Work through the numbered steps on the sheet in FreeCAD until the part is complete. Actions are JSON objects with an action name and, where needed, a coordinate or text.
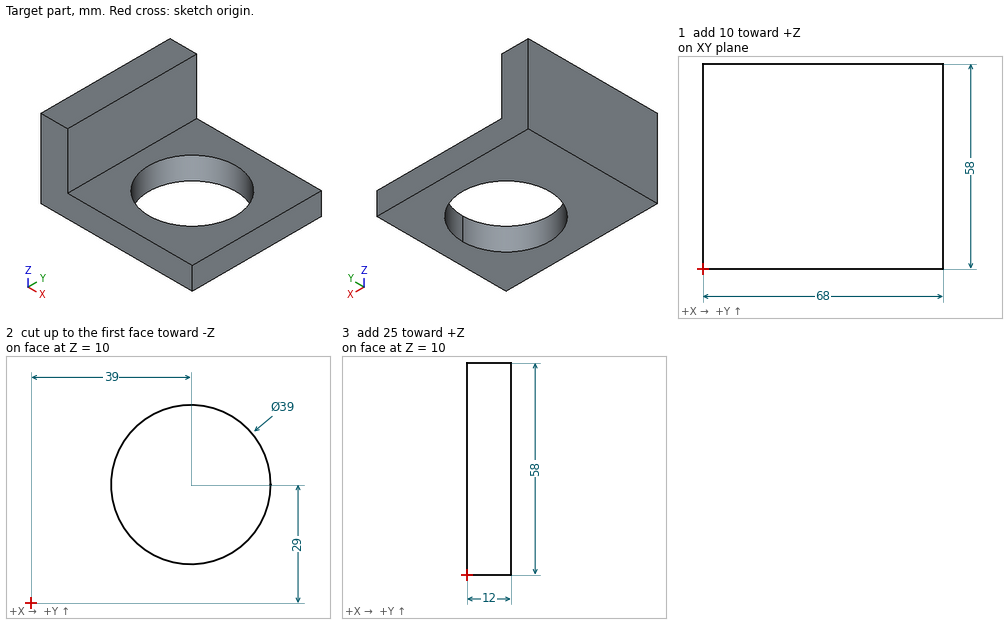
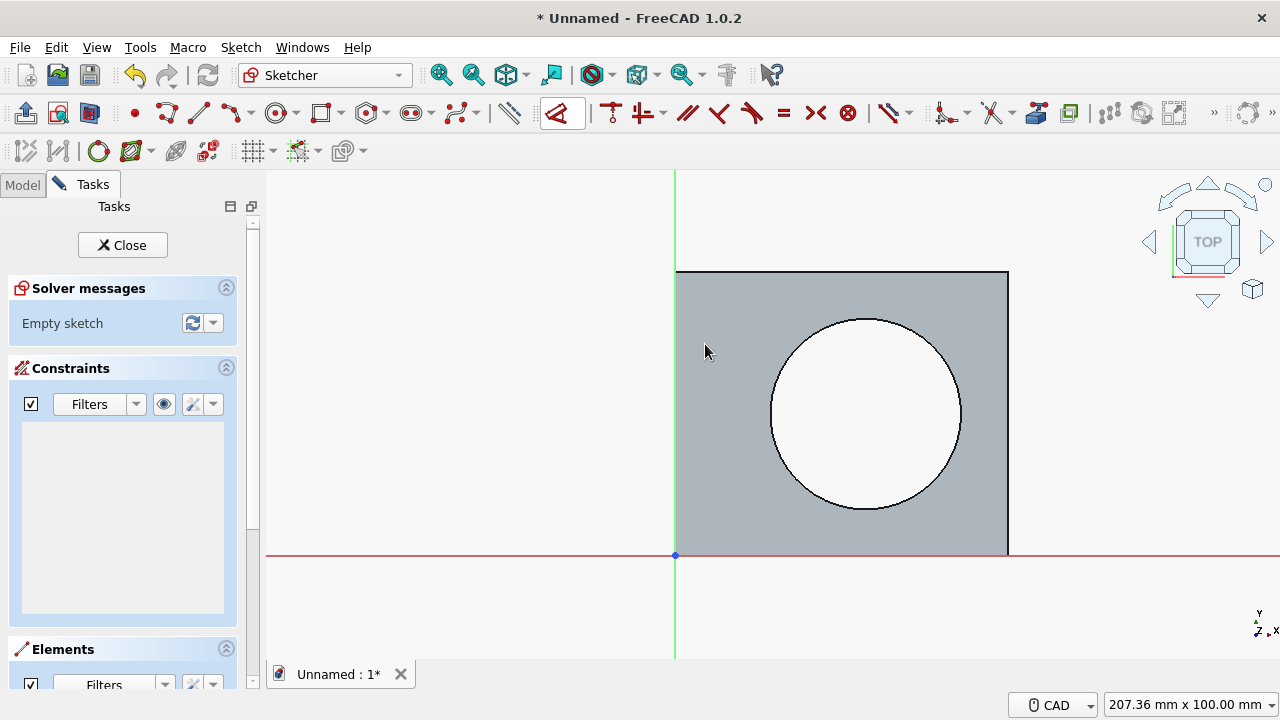
{"action": "key", "text": "g r"}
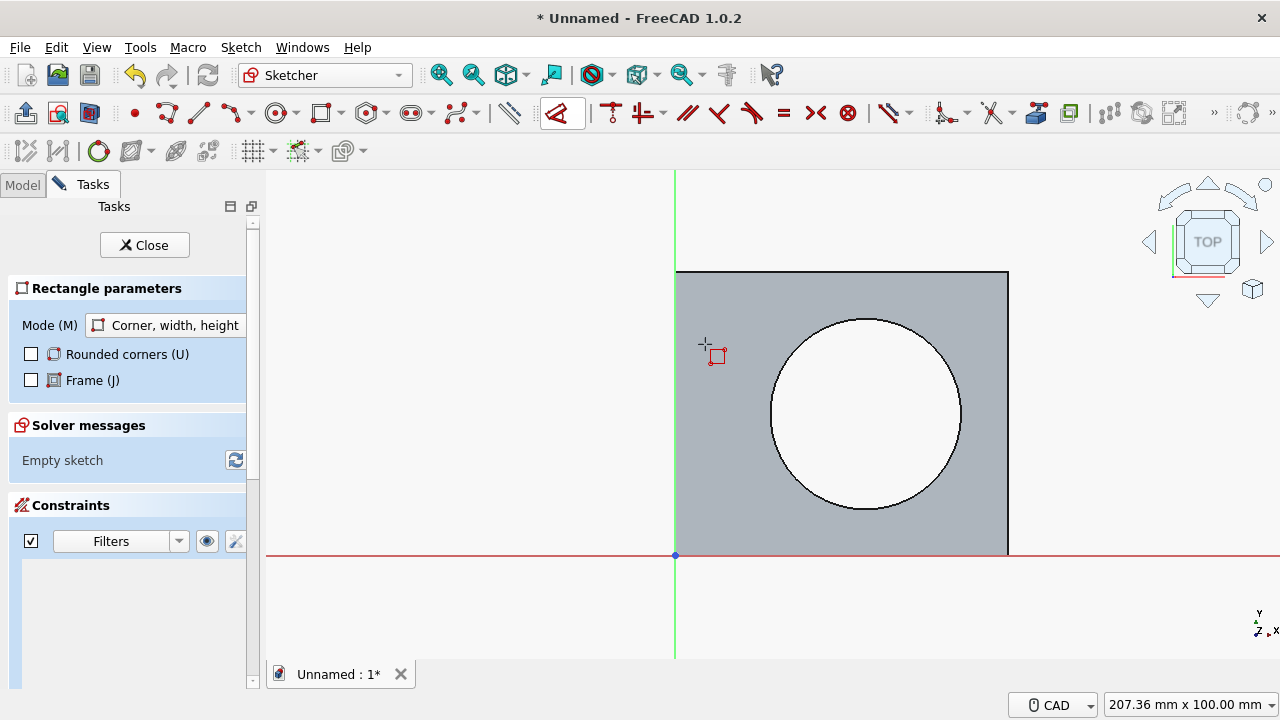
{"action": "left_click", "coordinate": [675, 556]}
{"action": "left_click", "coordinate": [734, 272]}
{"action": "key", "text": "Escape"}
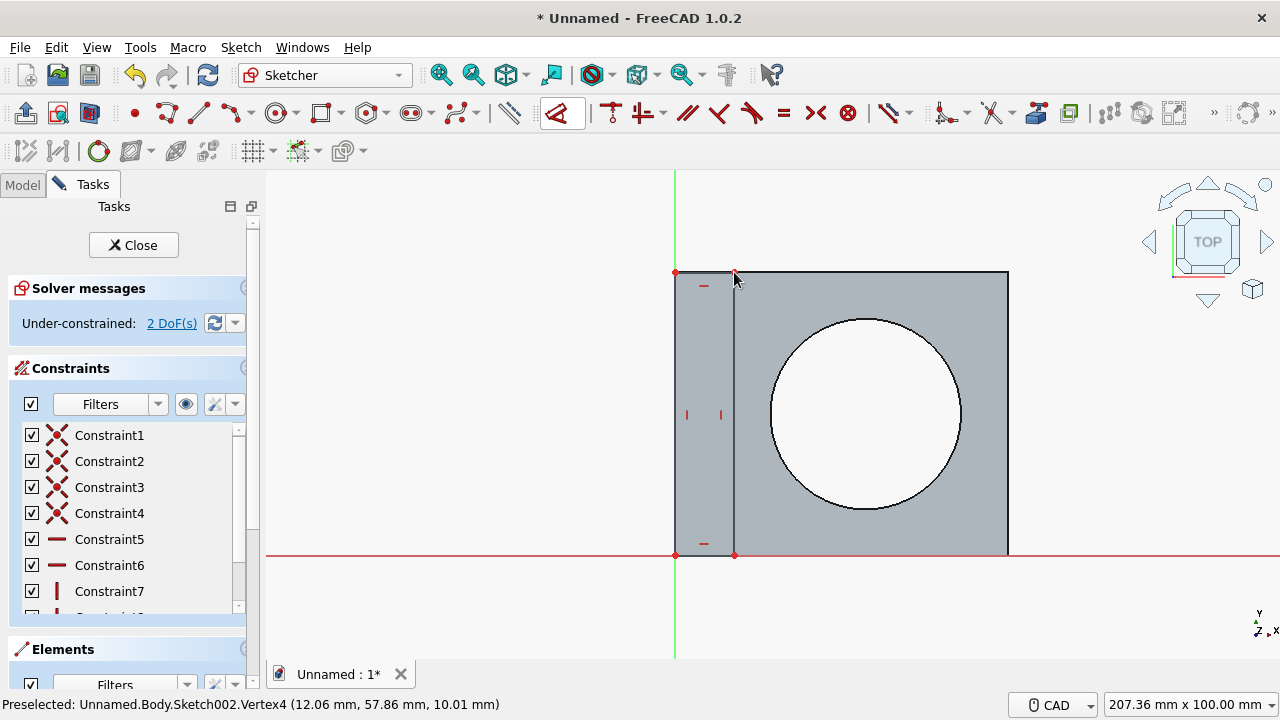
{"action": "left_click", "coordinate": [693, 556]}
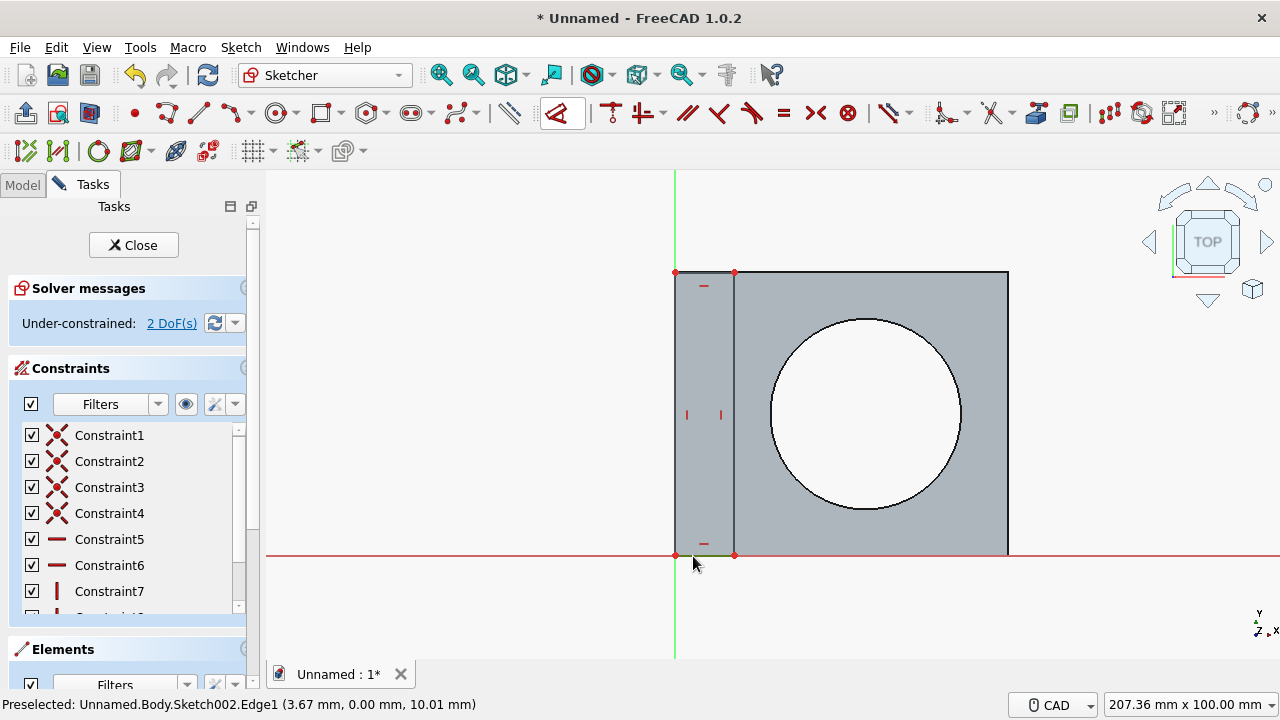
{"action": "key", "text": "l"}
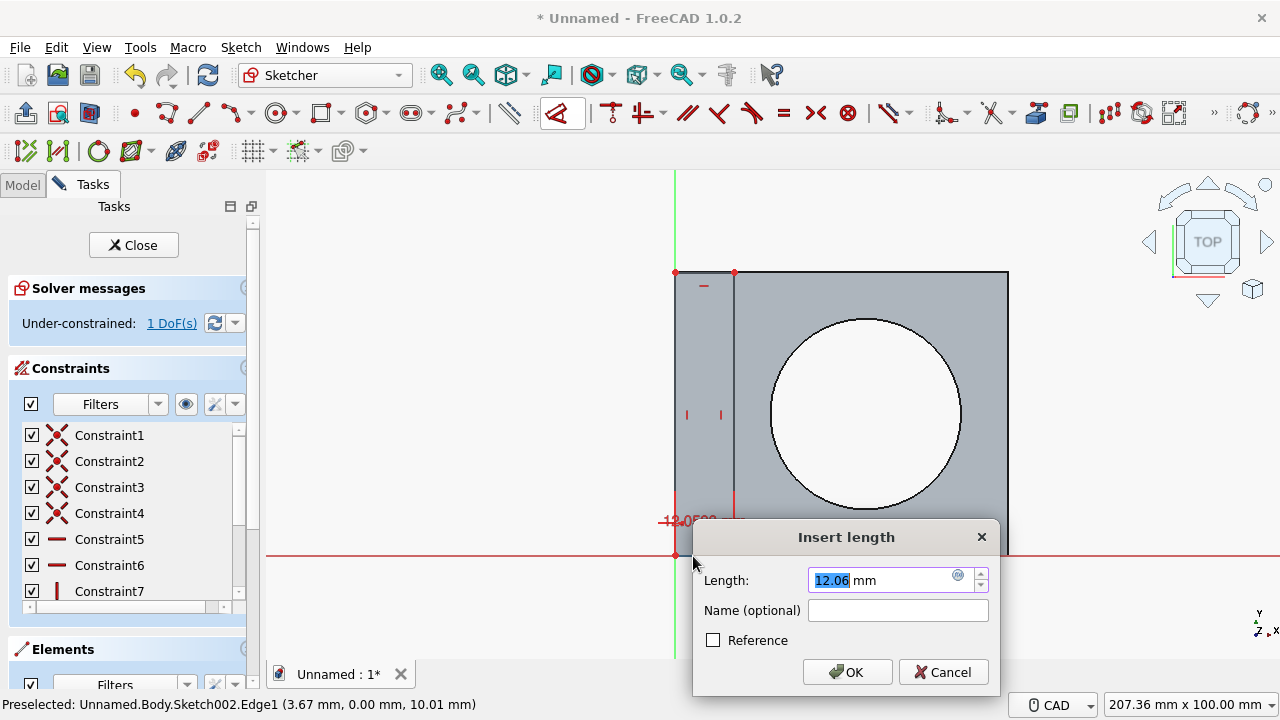
{"action": "type", "text": "12"}
{"action": "key", "text": "Return"}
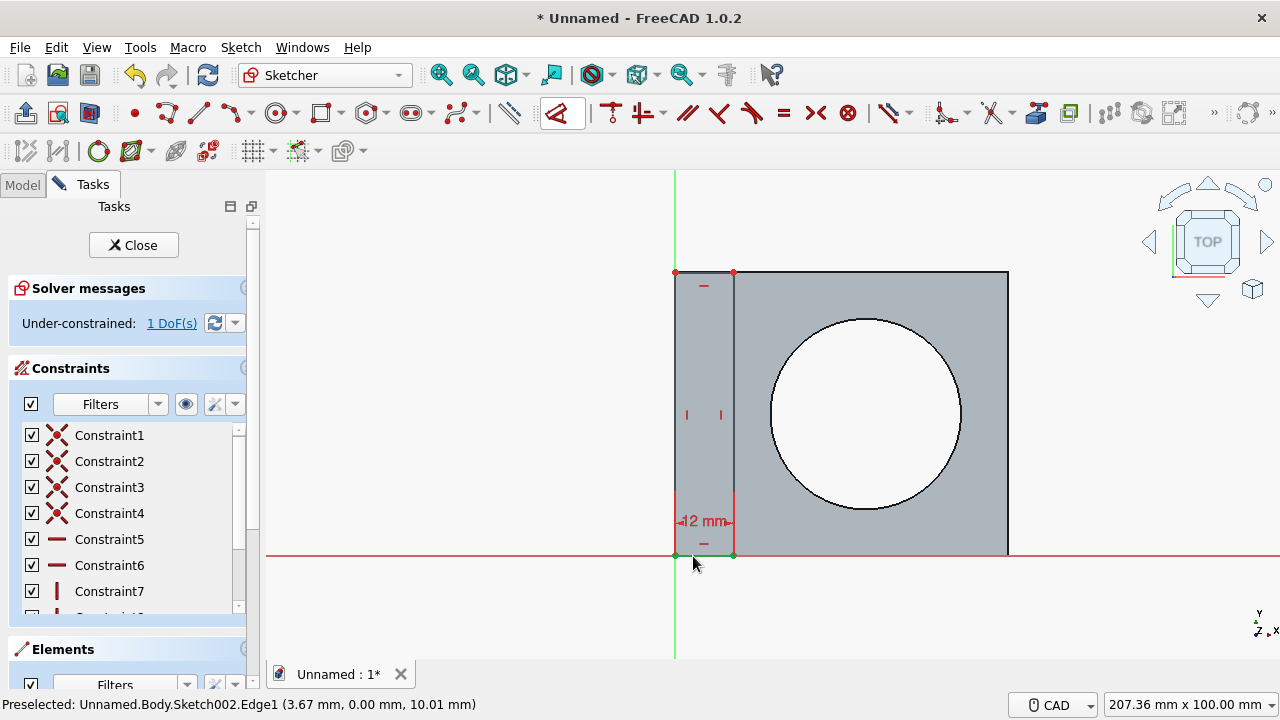
{"action": "left_click", "coordinate": [734, 471]}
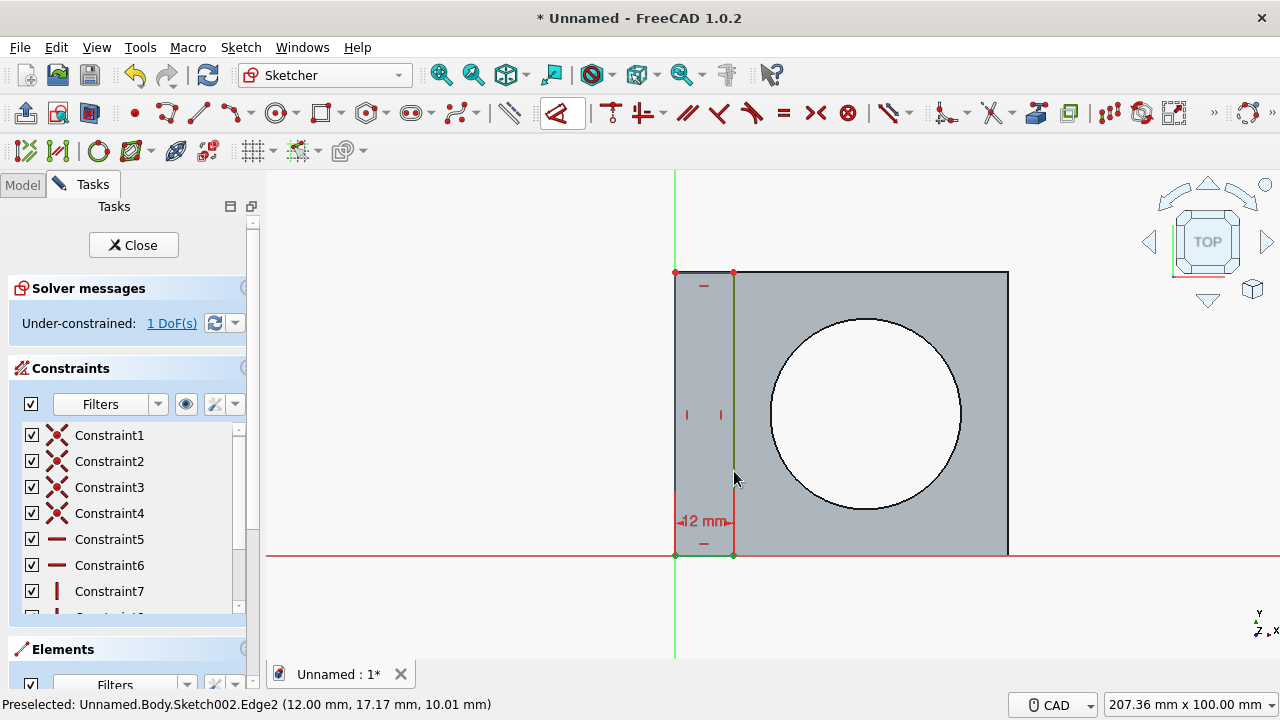
{"action": "key", "text": "i"}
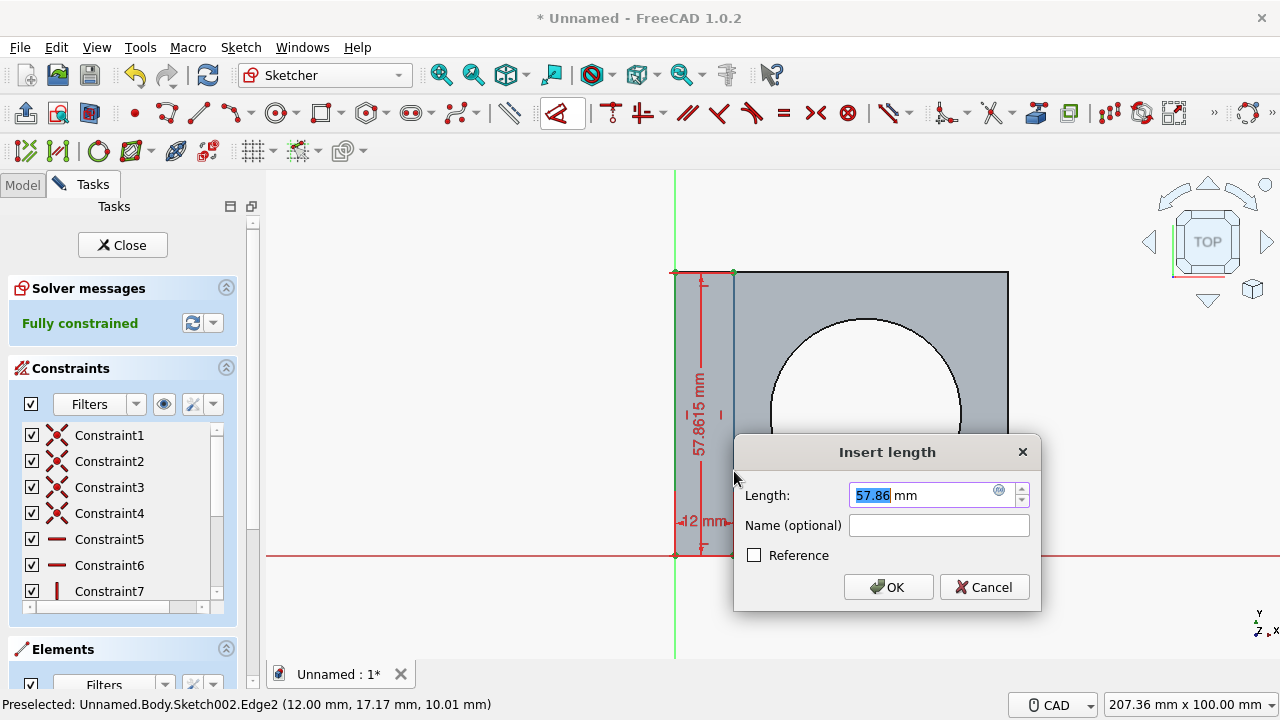
{"action": "type", "text": "58"}
{"action": "key", "text": "Return"}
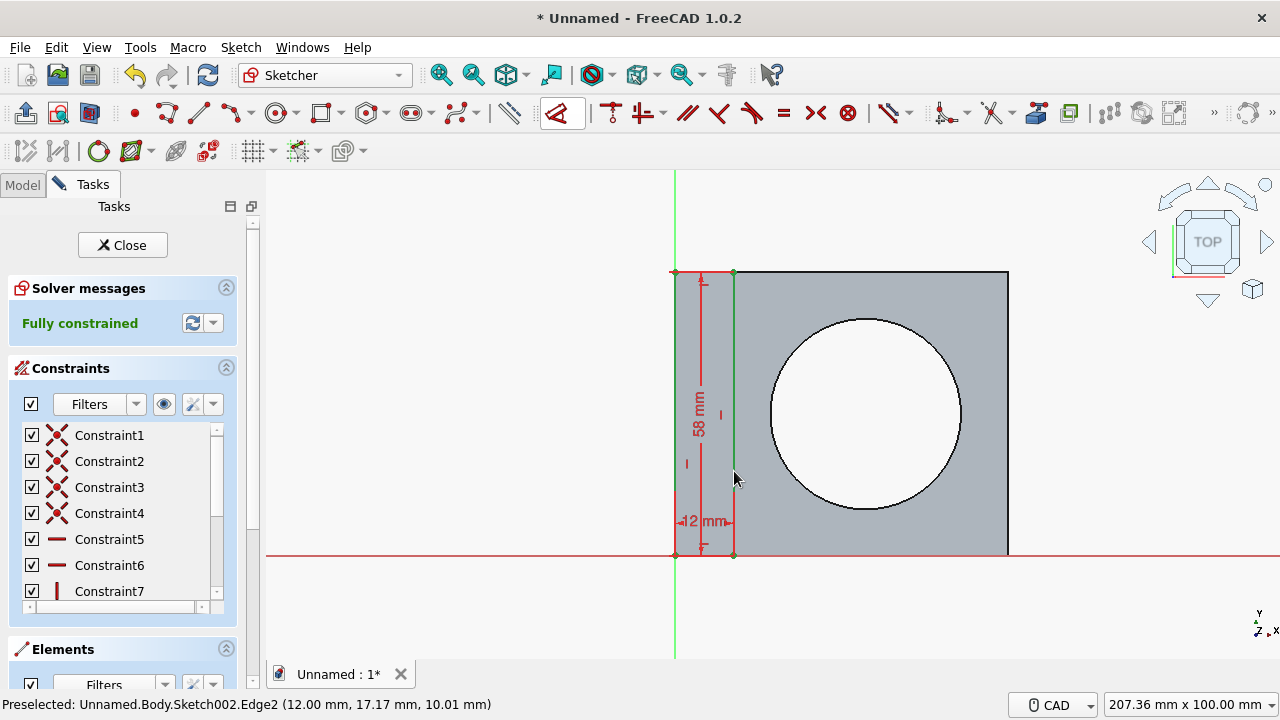
{"action": "left_click", "coordinate": [123, 245]}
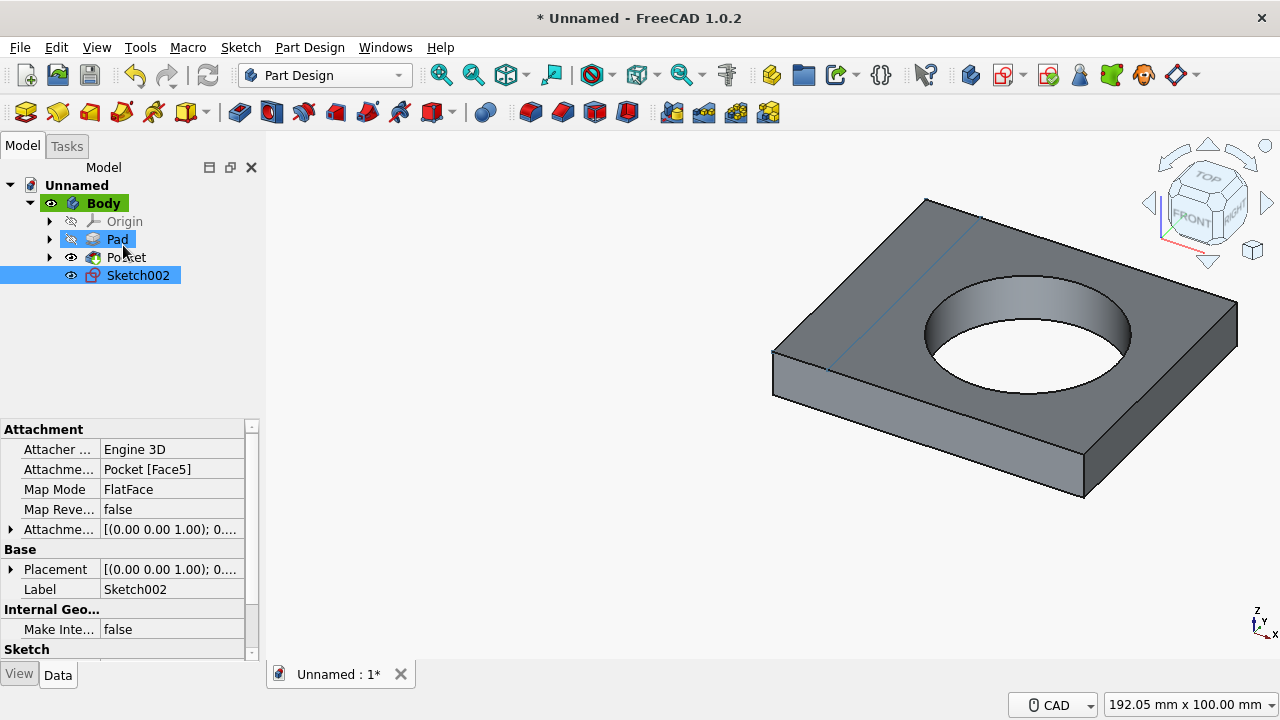
{"action": "left_click", "coordinate": [26, 112]}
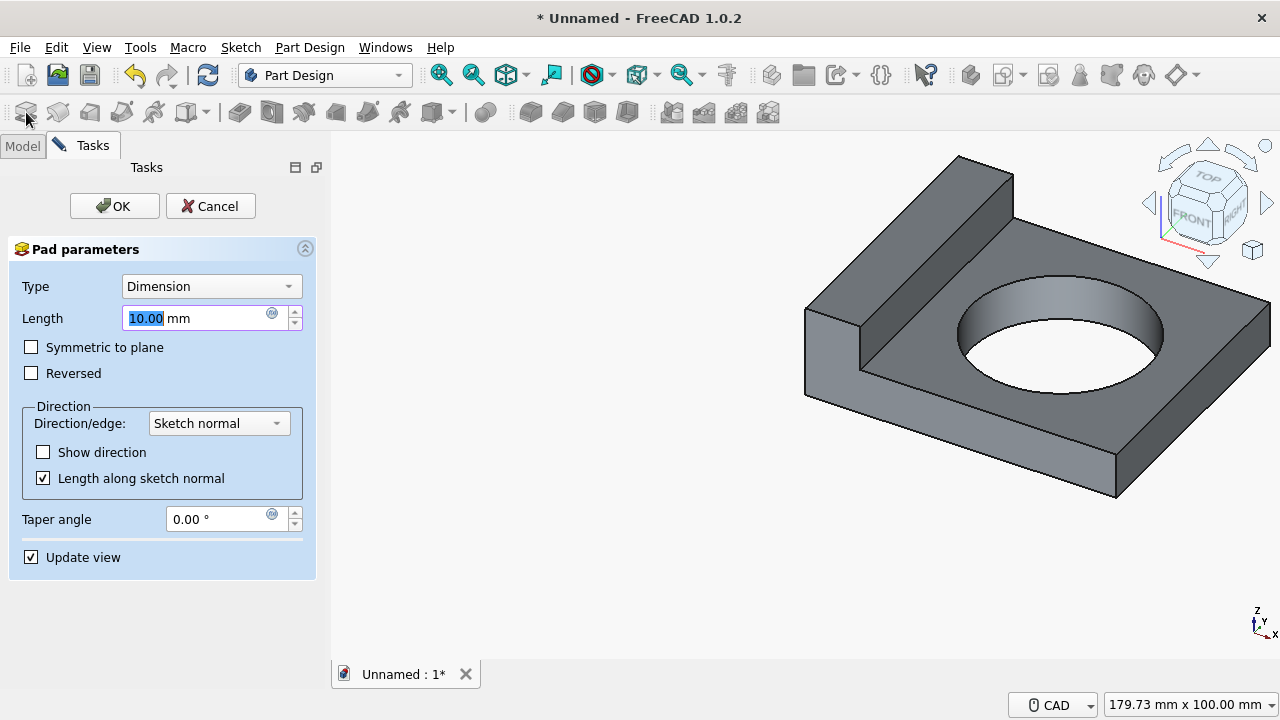
{"action": "type", "text": "25"}
{"action": "key", "text": "Tab"}